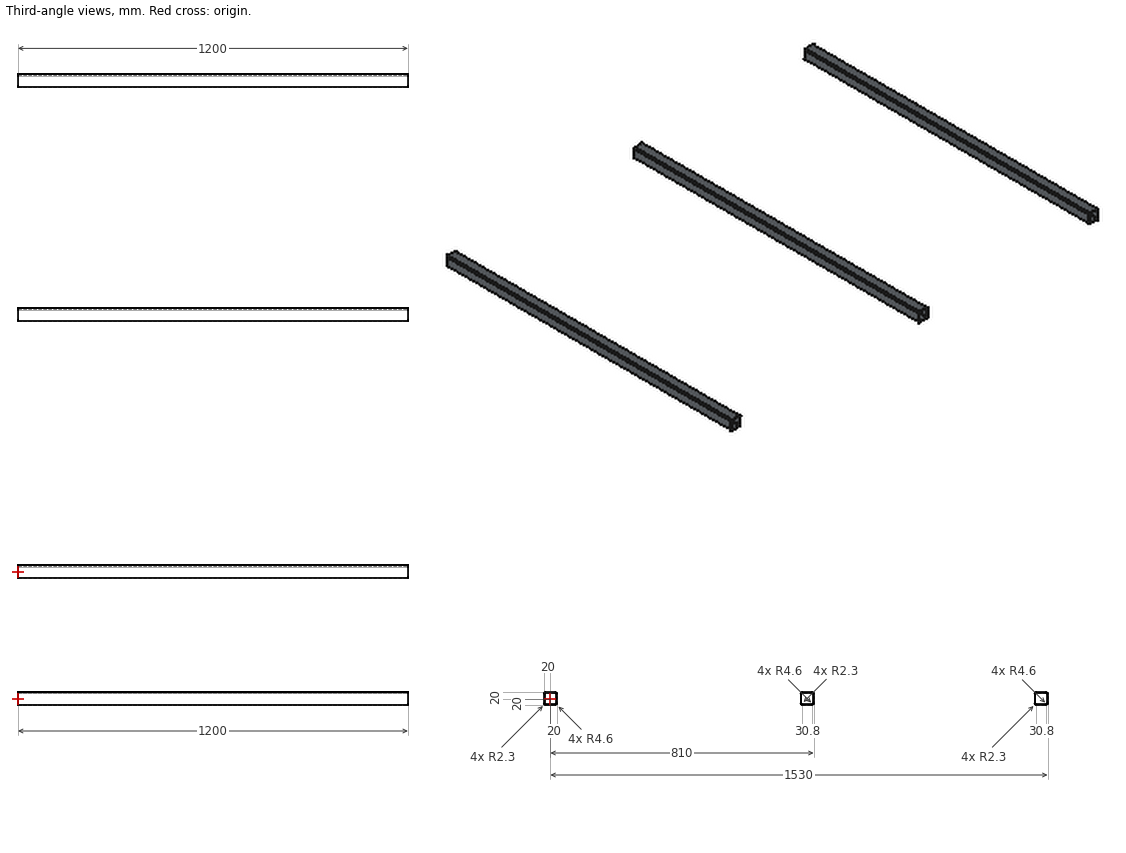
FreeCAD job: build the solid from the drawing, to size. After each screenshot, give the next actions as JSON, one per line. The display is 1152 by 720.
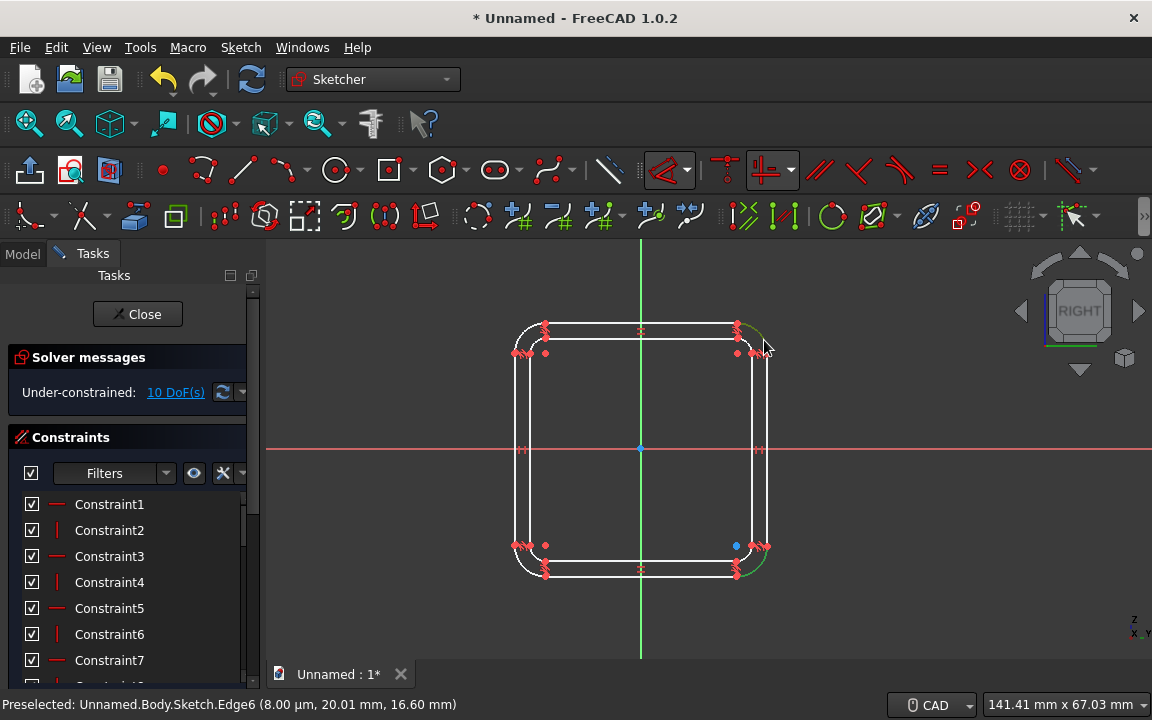
{"action": "left_click", "coordinate": [532, 327]}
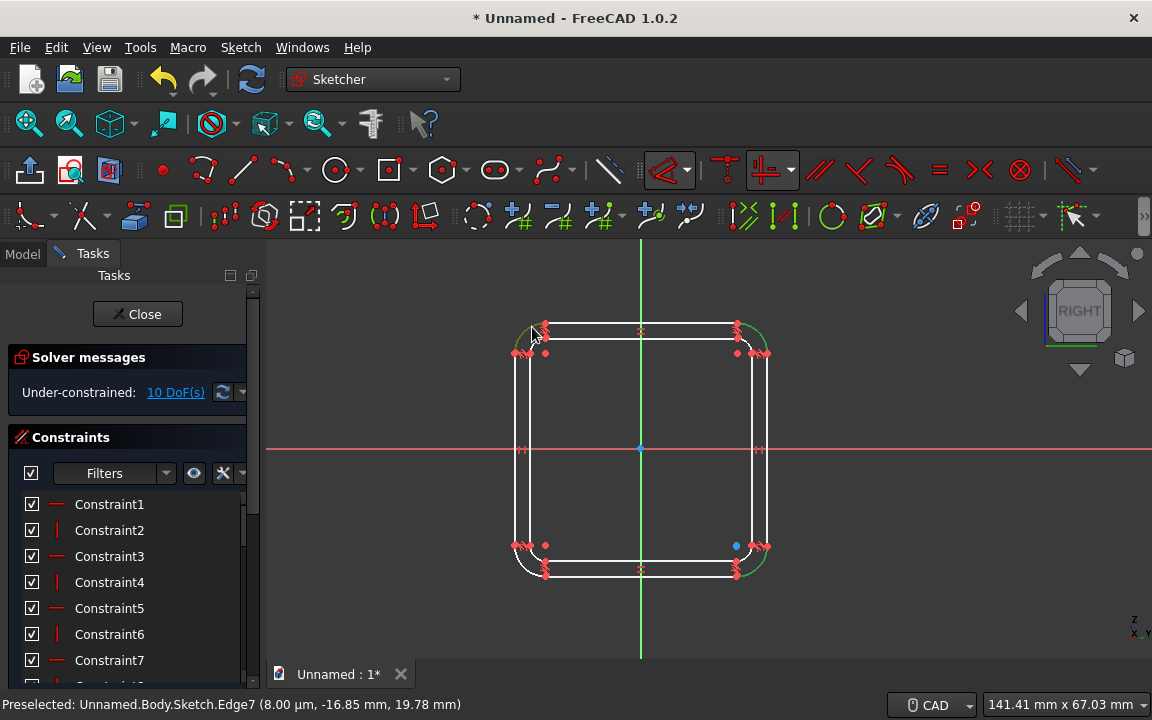
{"action": "left_click", "coordinate": [518, 560]}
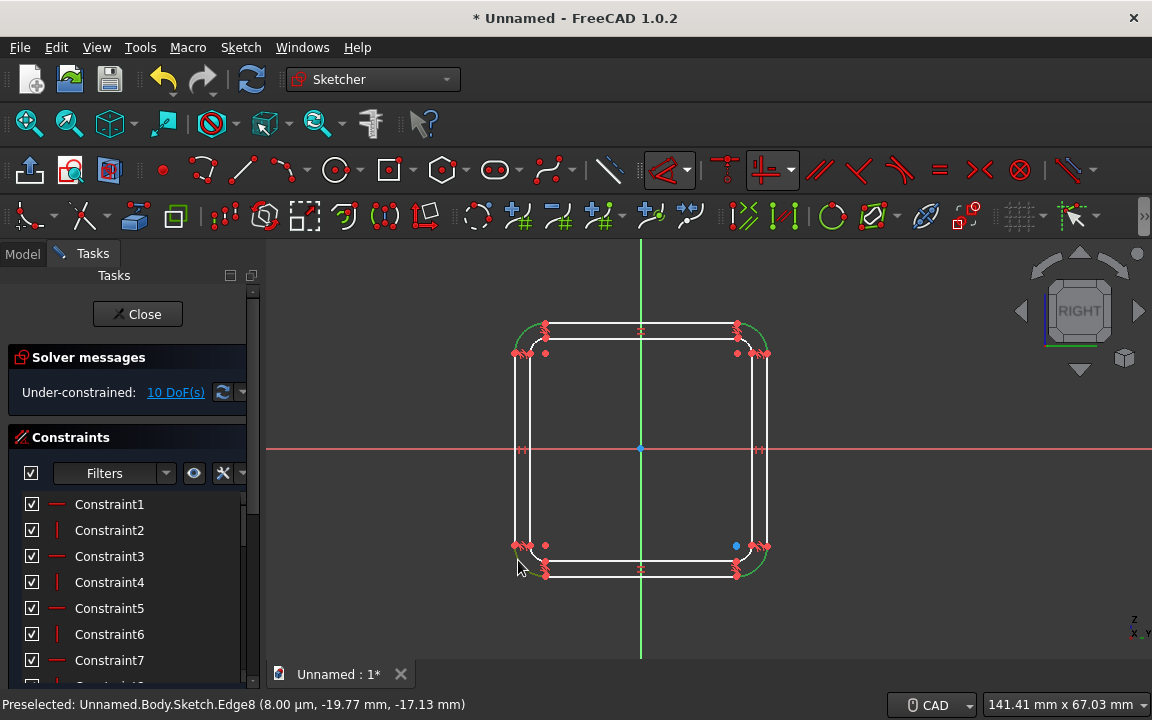
{"action": "left_click", "coordinate": [940, 170]}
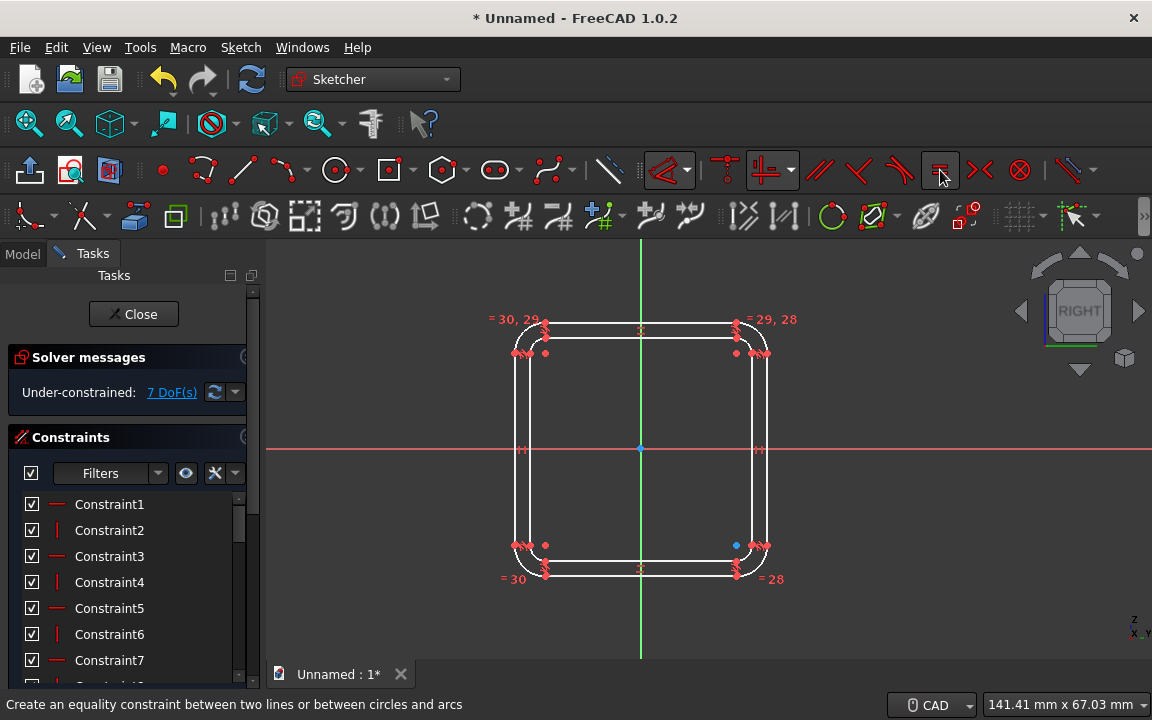
{"action": "left_click", "coordinate": [535, 557]}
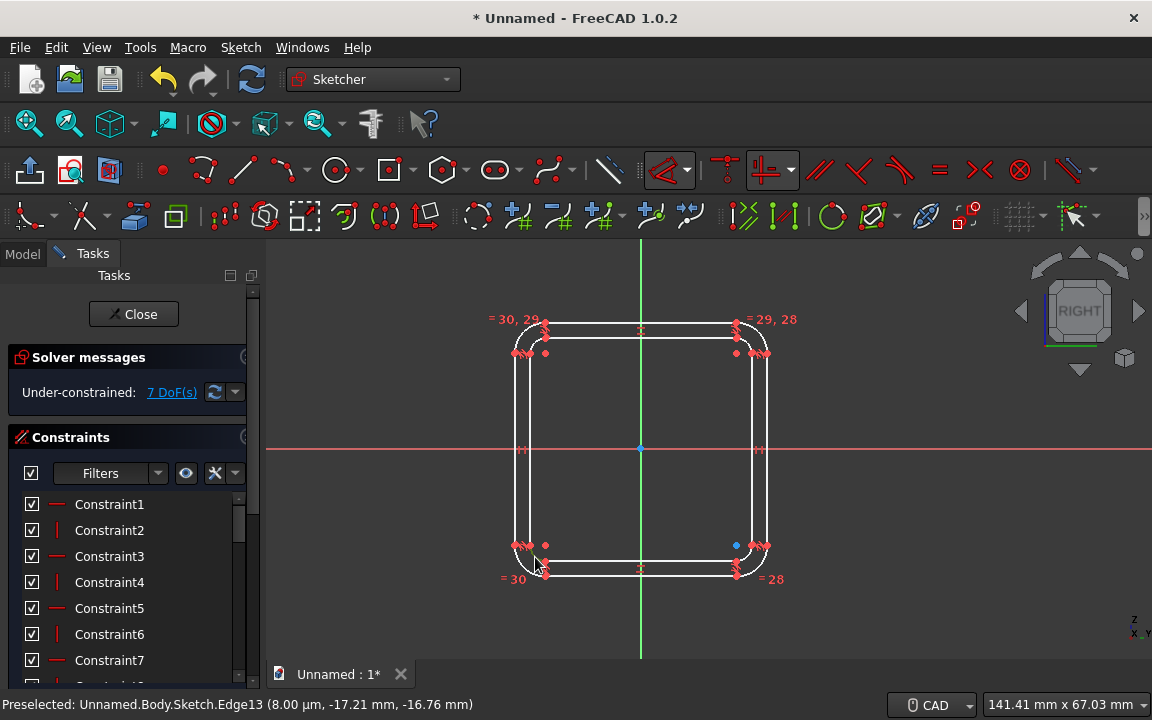
{"action": "left_click", "coordinate": [747, 557]}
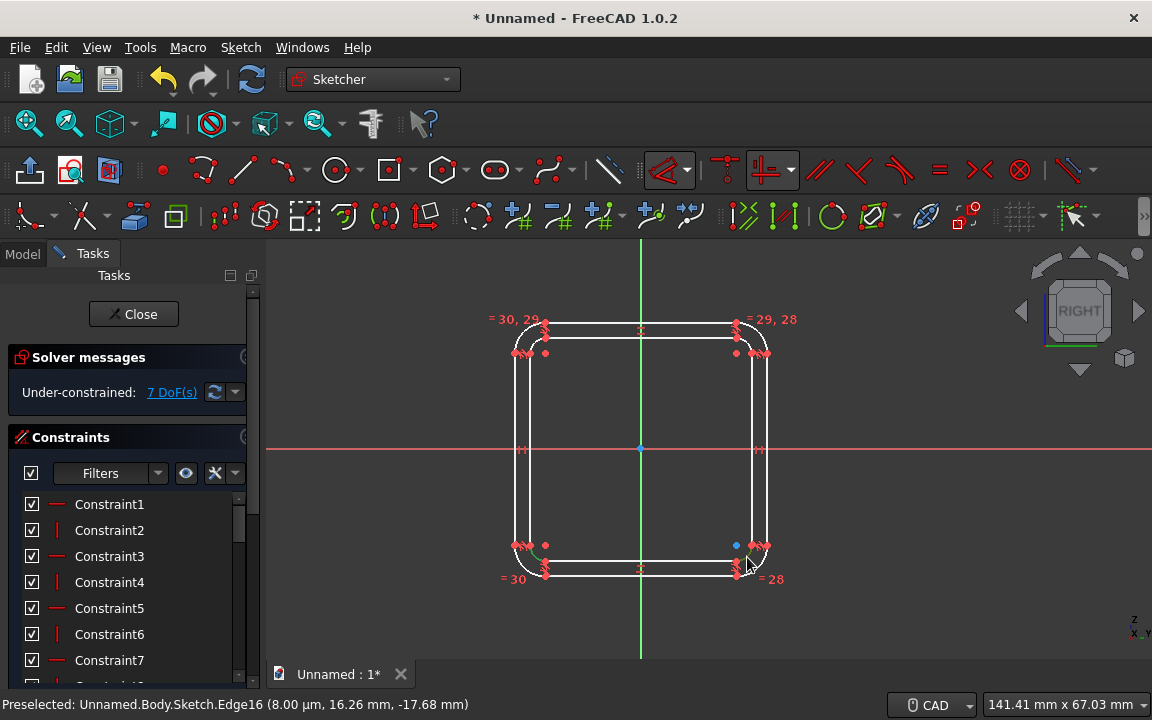
{"action": "key", "text": "e"}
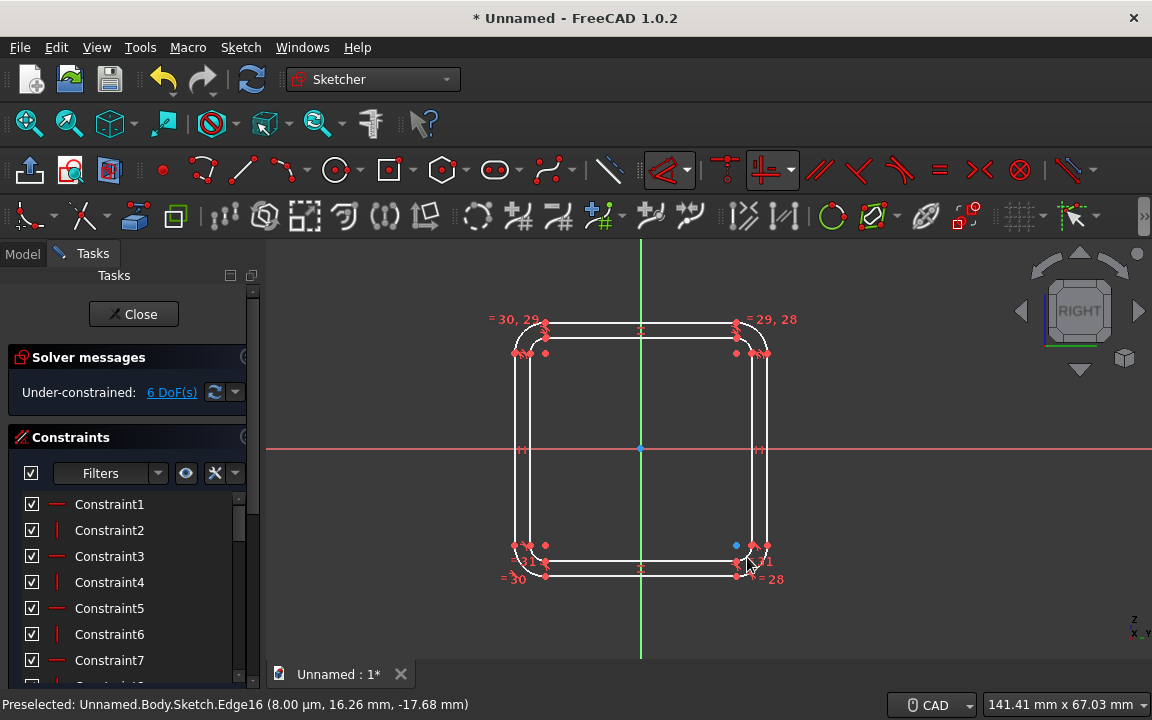
{"action": "left_click", "coordinate": [664, 170]}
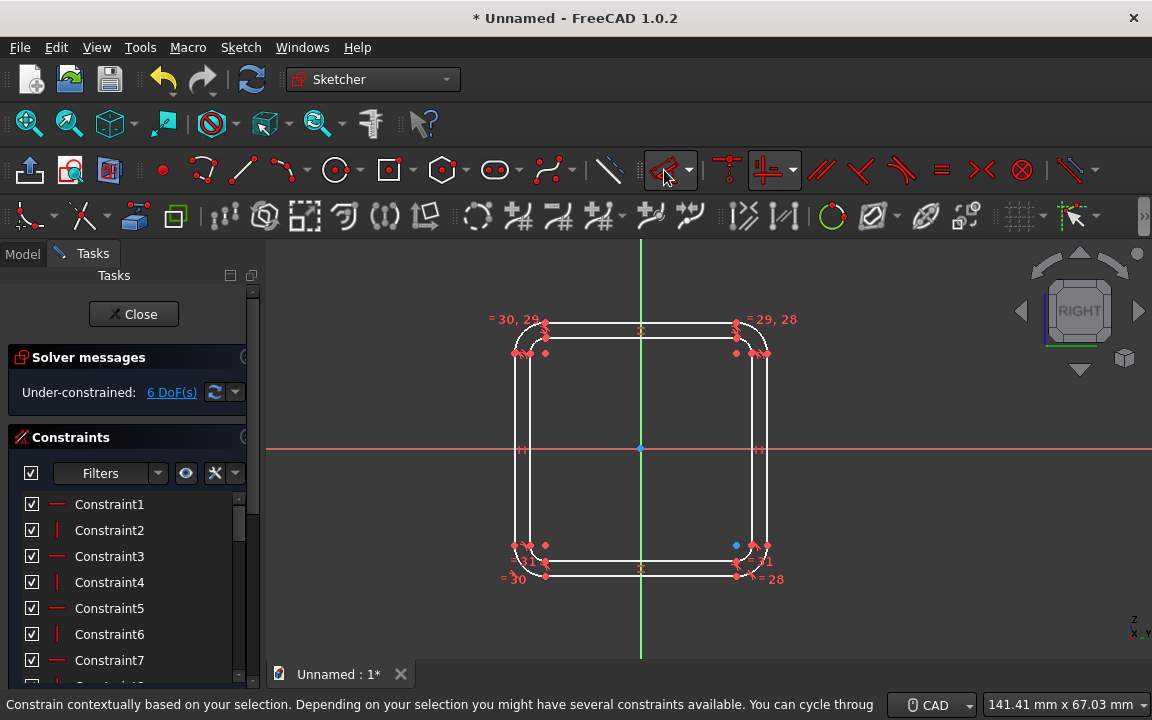
{"action": "scroll", "coordinate": [750, 573], "scroll_direction": "up", "scroll_amount": 2}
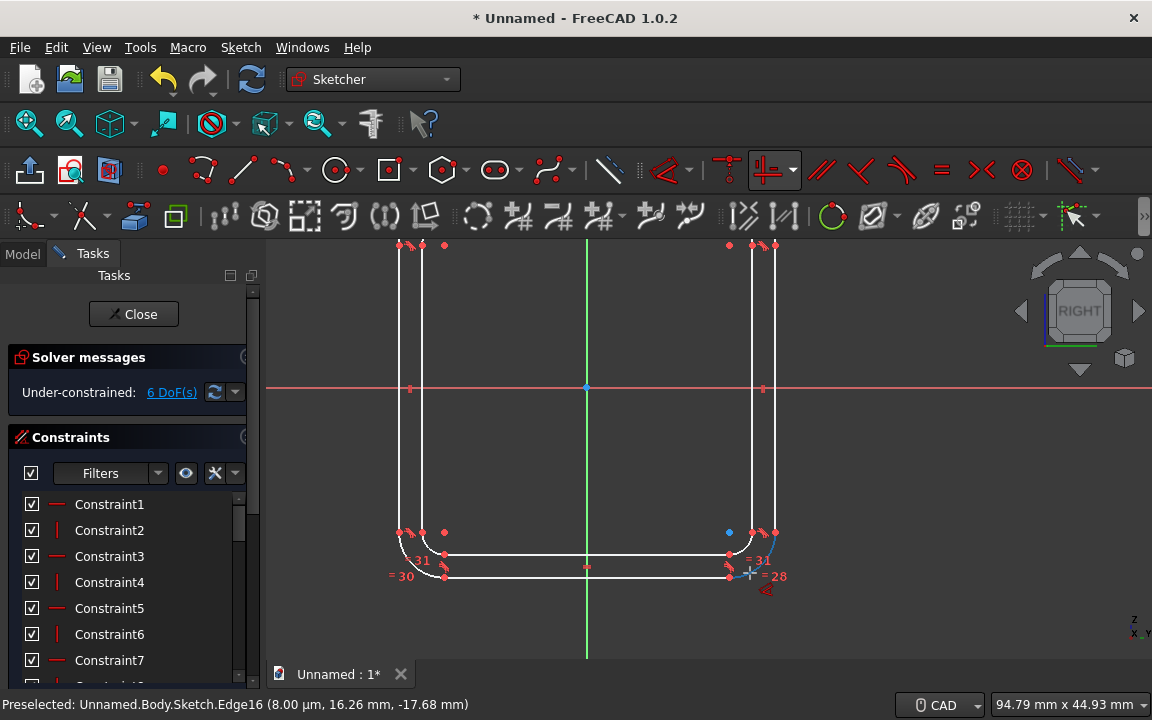
{"action": "left_click", "coordinate": [750, 573]}
{"action": "left_click", "coordinate": [764, 602]}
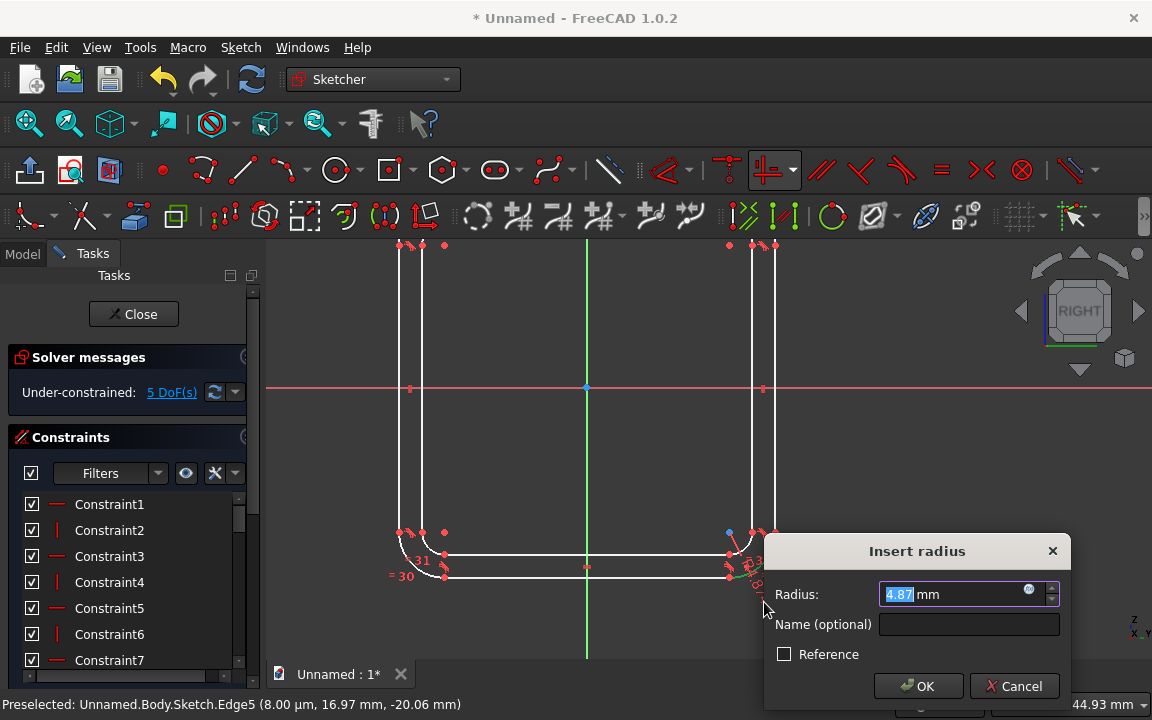
{"action": "type", "text": "4.6"}
{"action": "key", "text": "Return"}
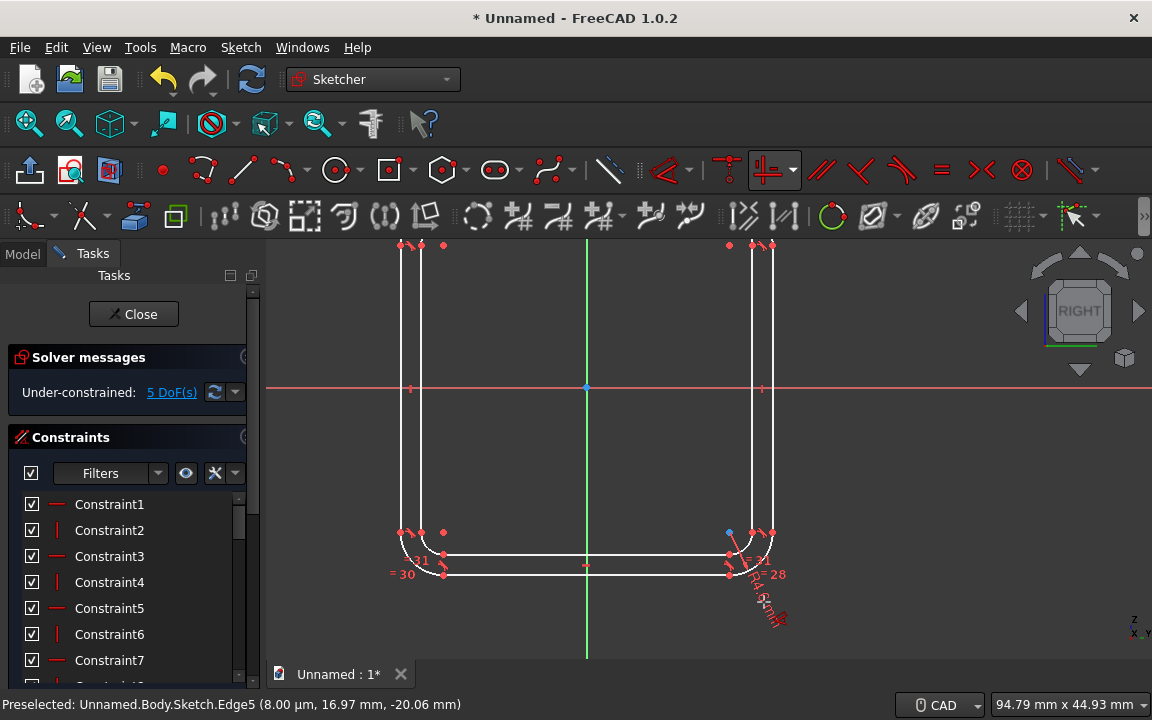
{"action": "scroll", "coordinate": [424, 542], "scroll_direction": "up", "scroll_amount": 4}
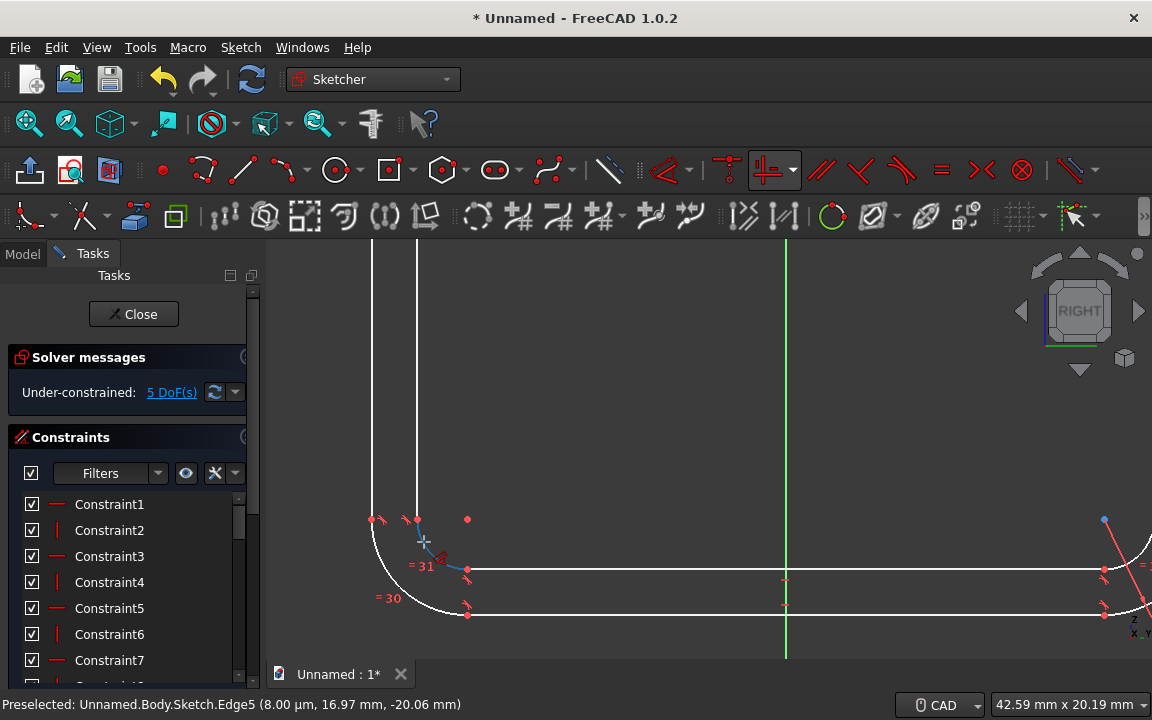
{"action": "left_click", "coordinate": [423, 542]}
{"action": "left_click", "coordinate": [394, 557]}